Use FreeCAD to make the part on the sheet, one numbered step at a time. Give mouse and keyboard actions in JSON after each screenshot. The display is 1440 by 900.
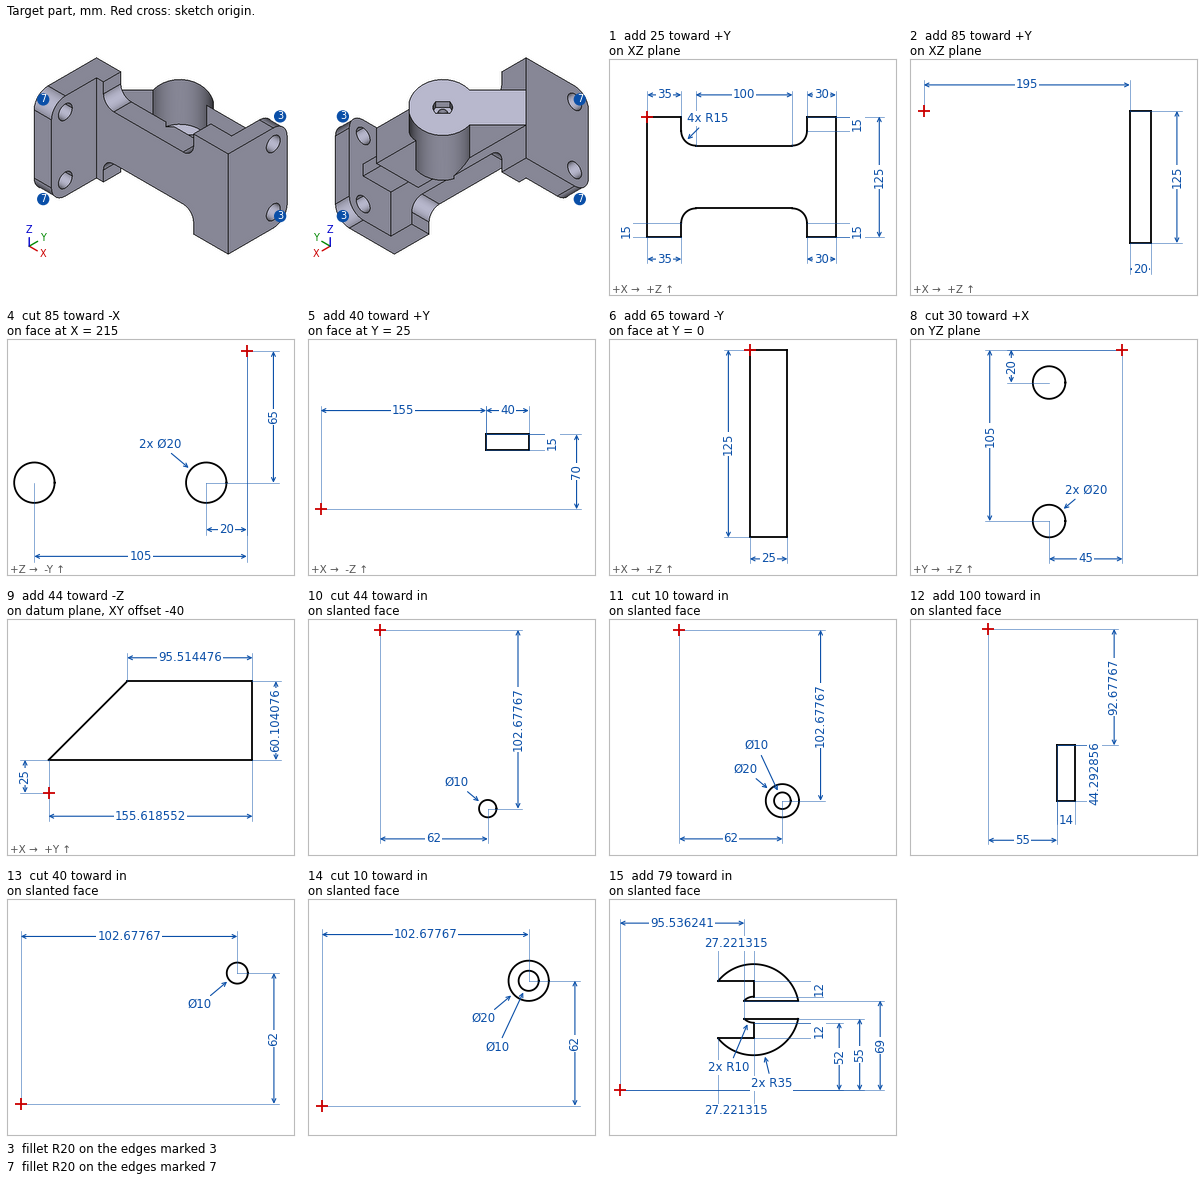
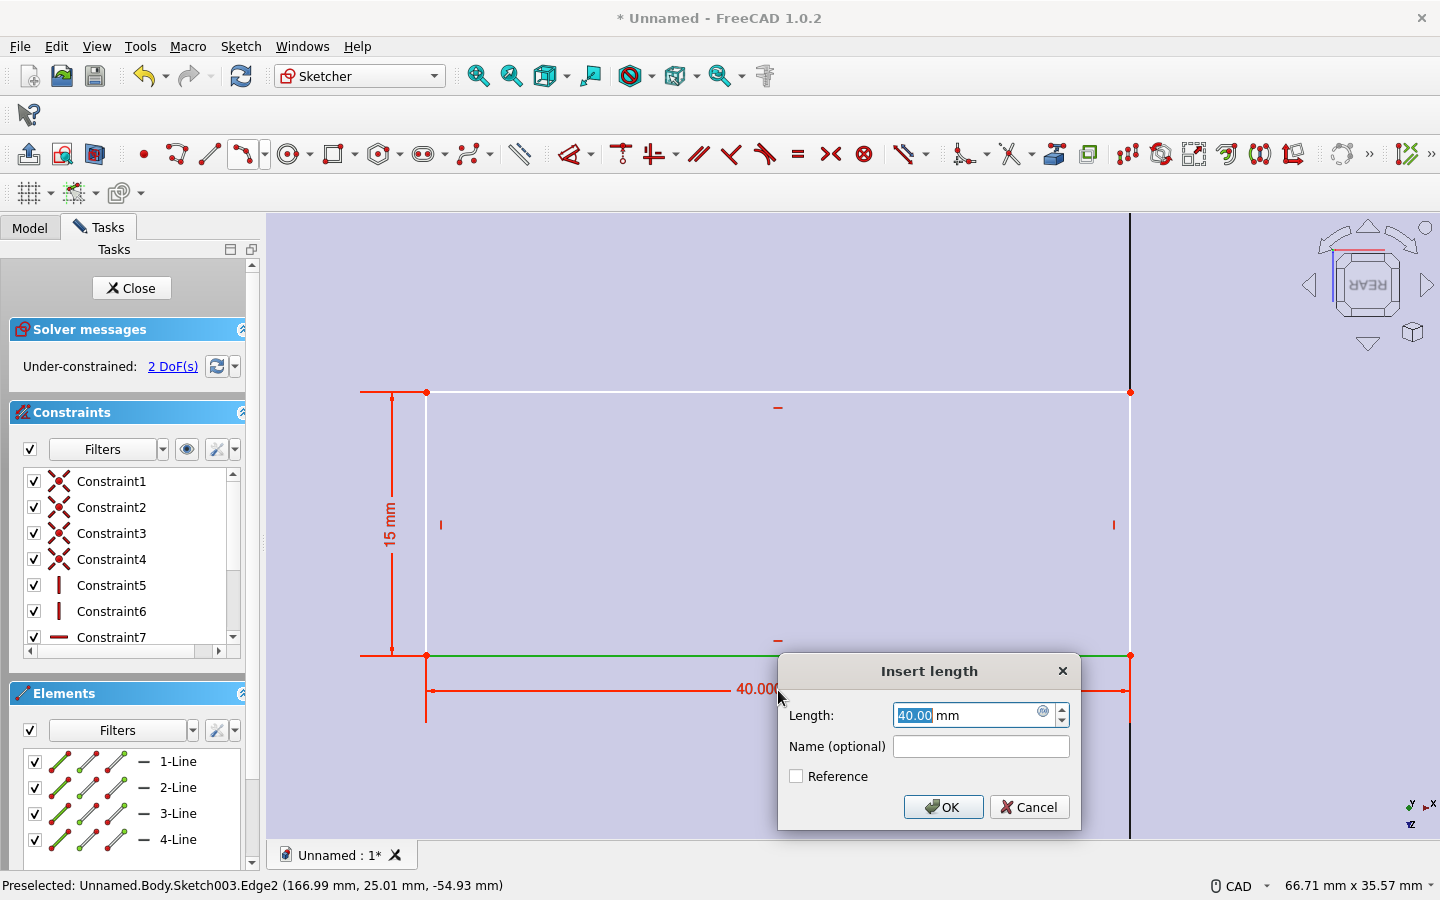
{"action": "type", "text": "40"}
{"action": "key", "text": "Return"}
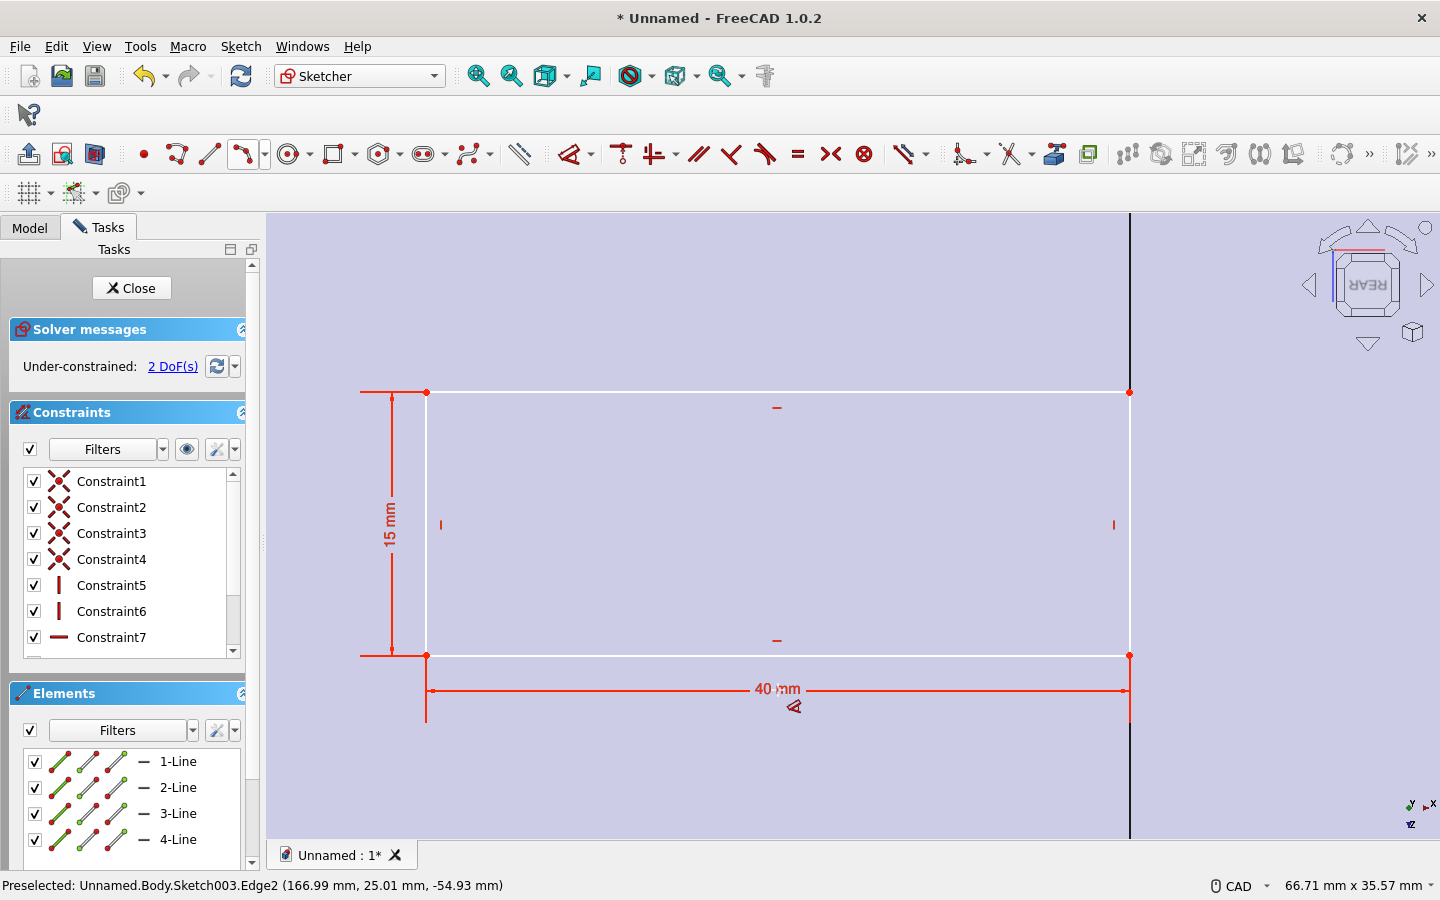
{"action": "left_click", "coordinate": [426, 392]}
{"action": "left_click", "coordinate": [460, 602]}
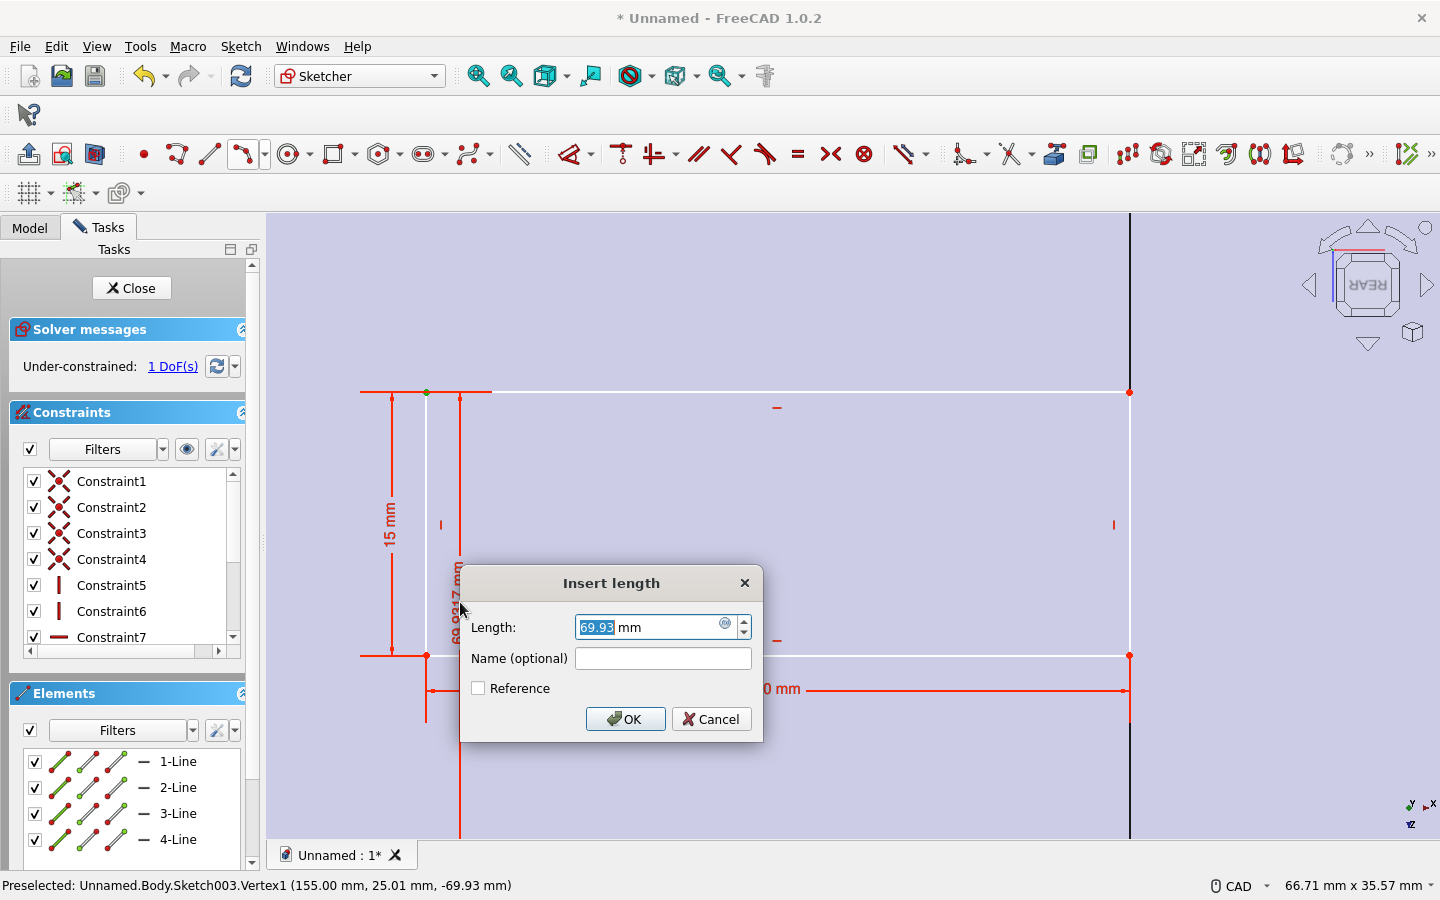
{"action": "type", "text": "70"}
{"action": "key", "text": "Return"}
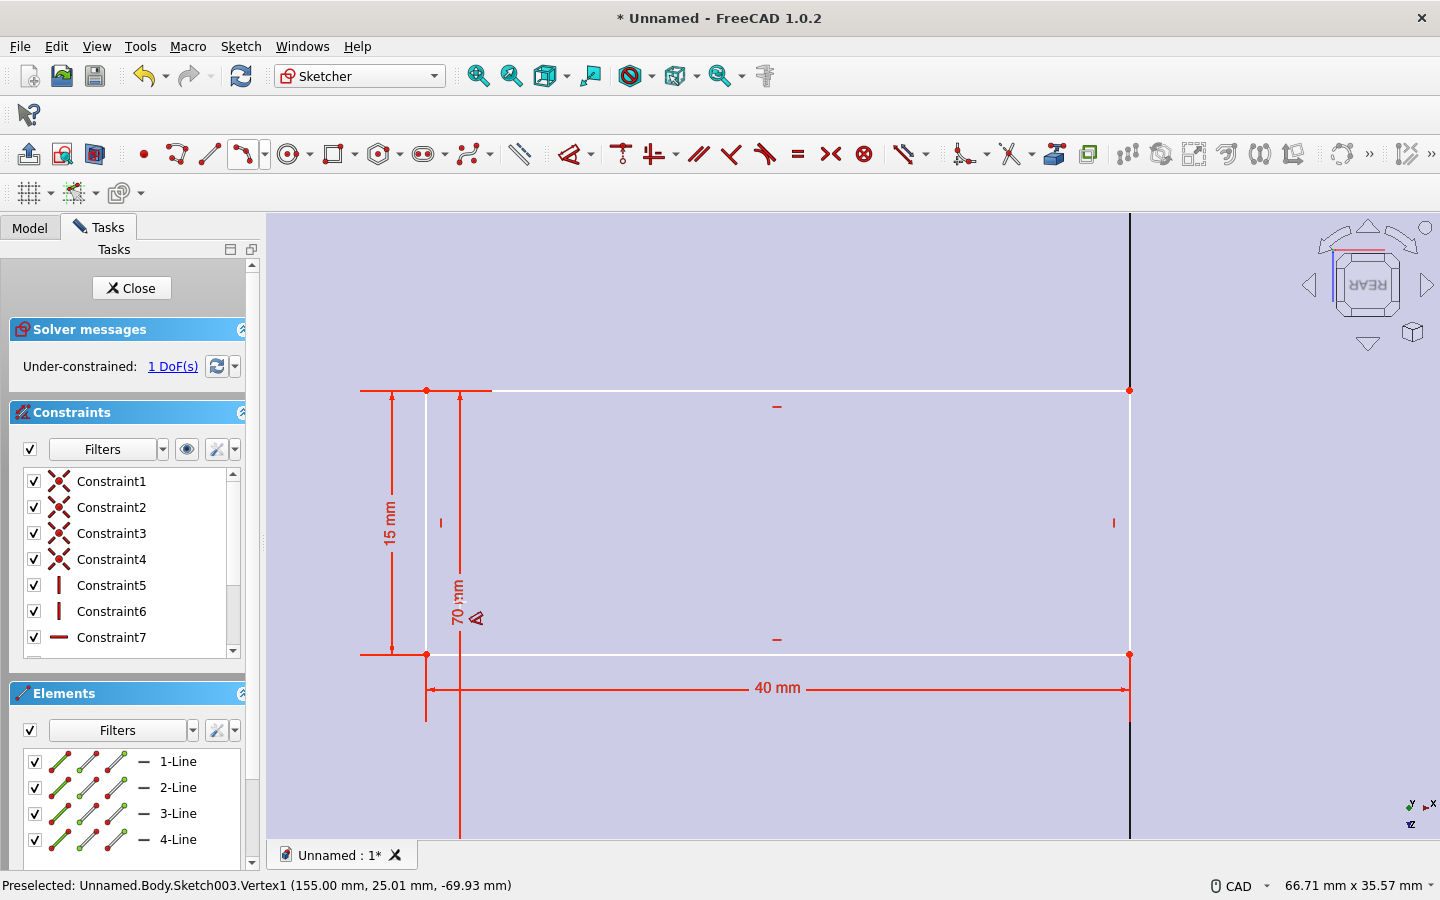
{"action": "left_click", "coordinate": [426, 391]}
{"action": "left_click", "coordinate": [360, 357]}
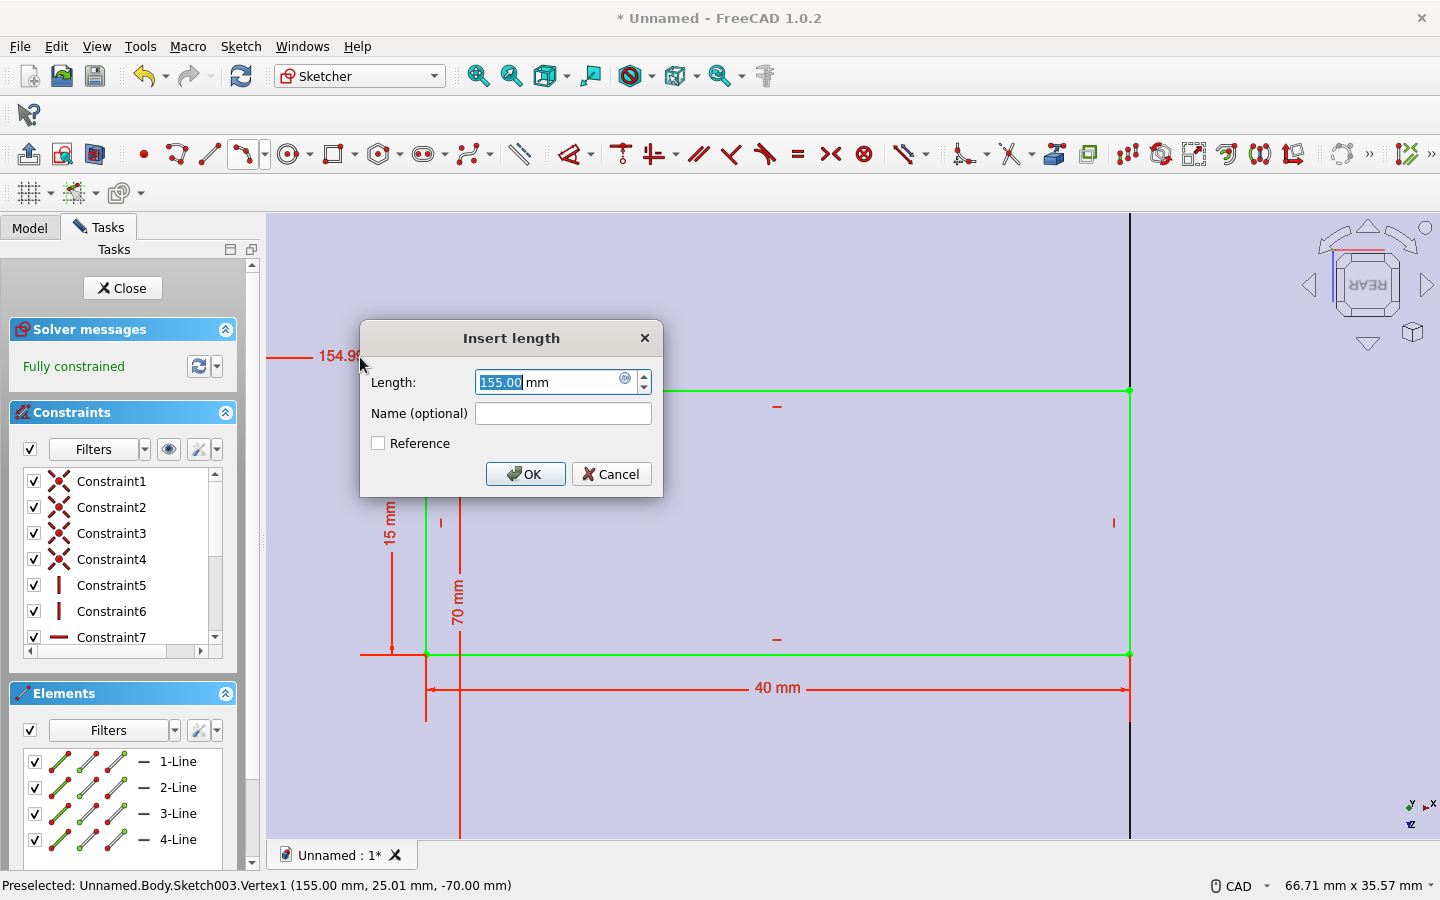
{"action": "type", "text": "155"}
{"action": "key", "text": "Return"}
{"action": "key", "text": "Escape"}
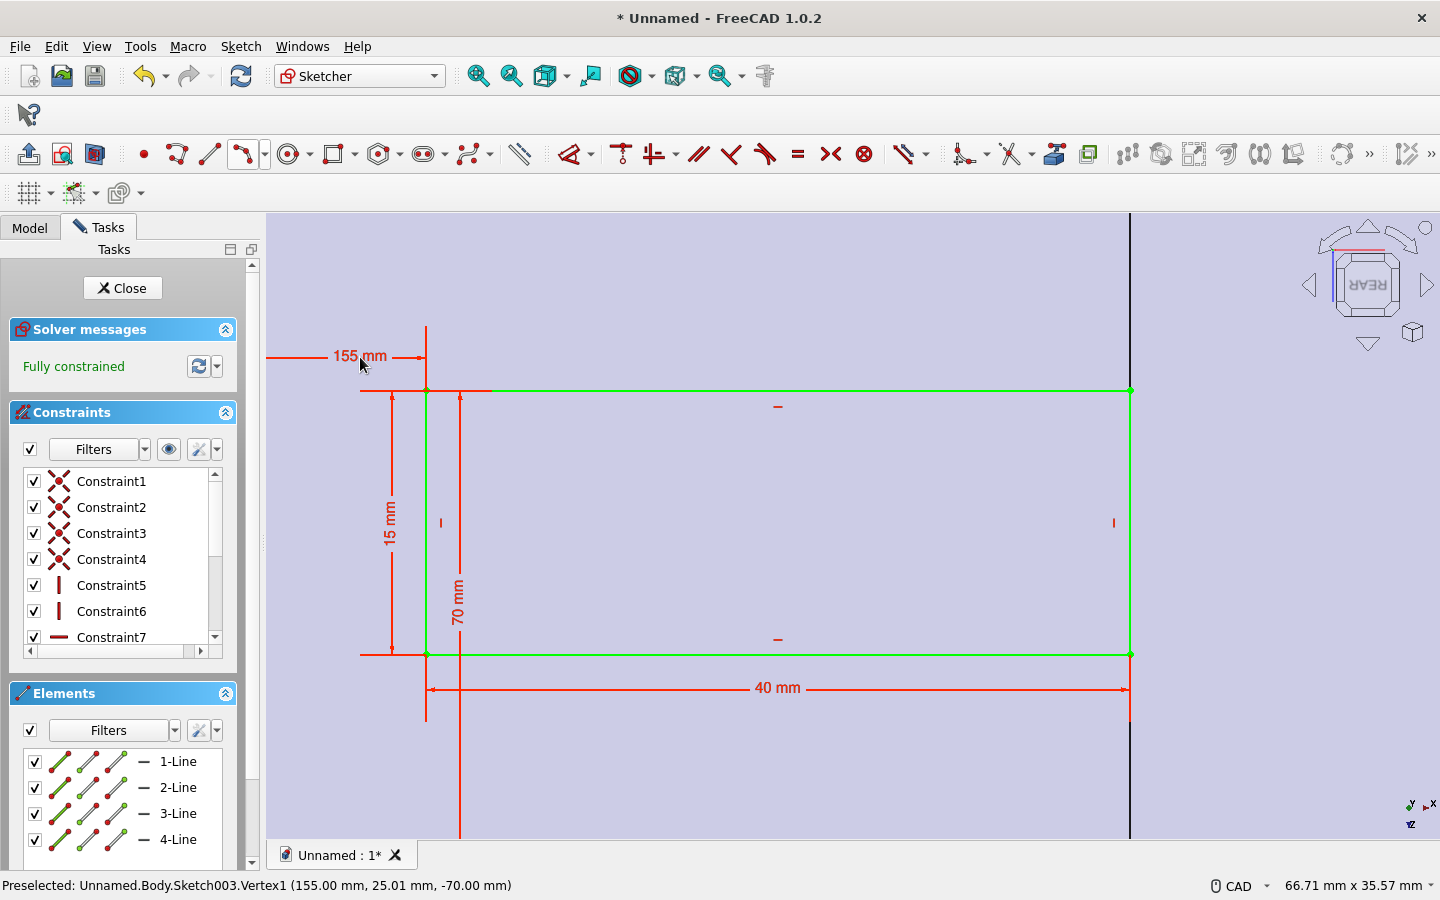
{"action": "left_click", "coordinate": [123, 288]}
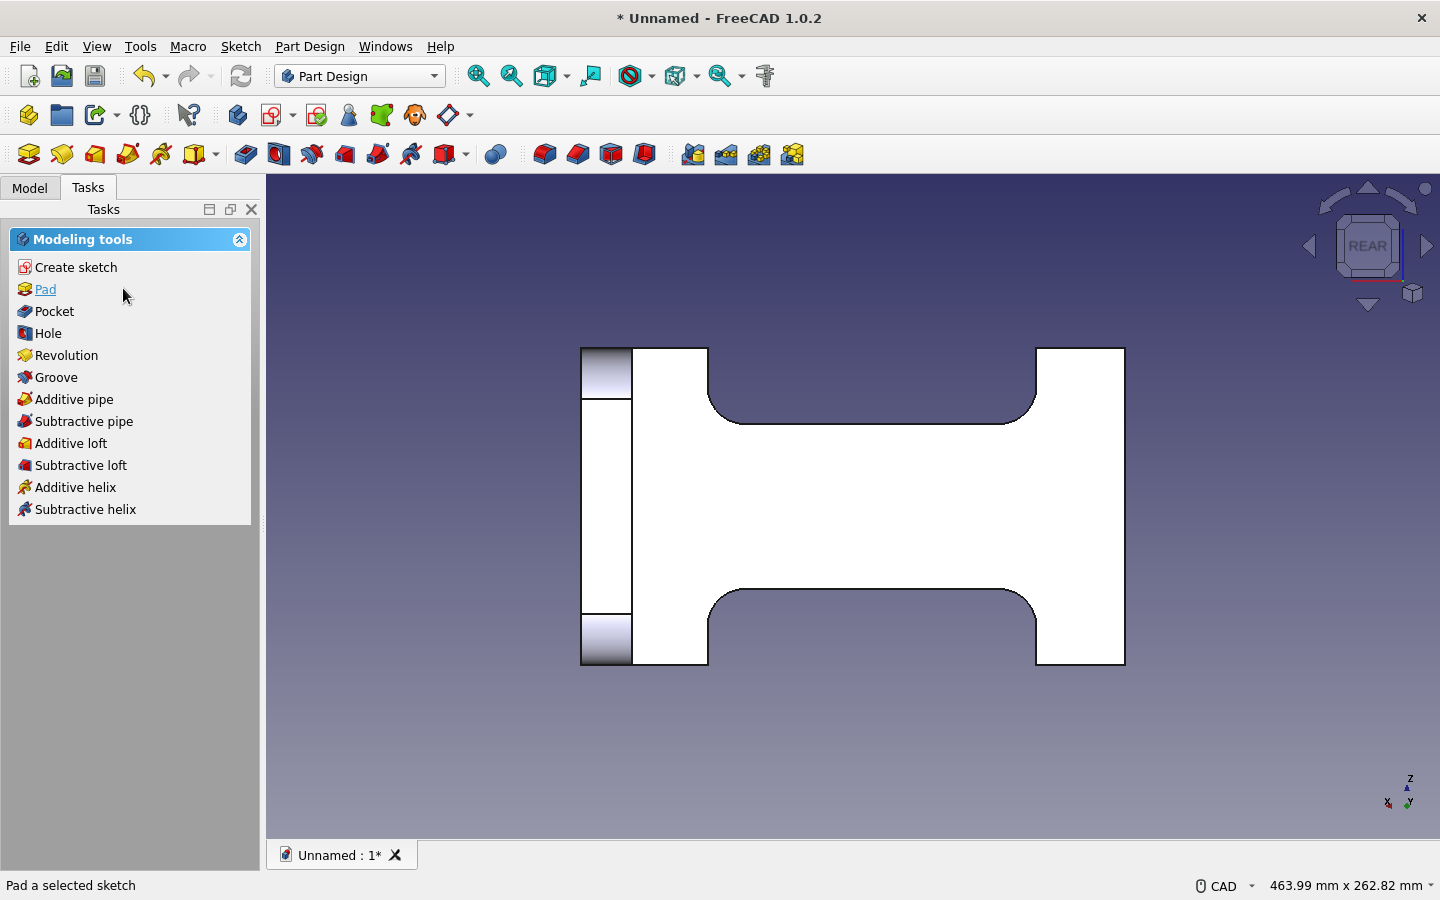
{"action": "left_click", "coordinate": [29, 154]}